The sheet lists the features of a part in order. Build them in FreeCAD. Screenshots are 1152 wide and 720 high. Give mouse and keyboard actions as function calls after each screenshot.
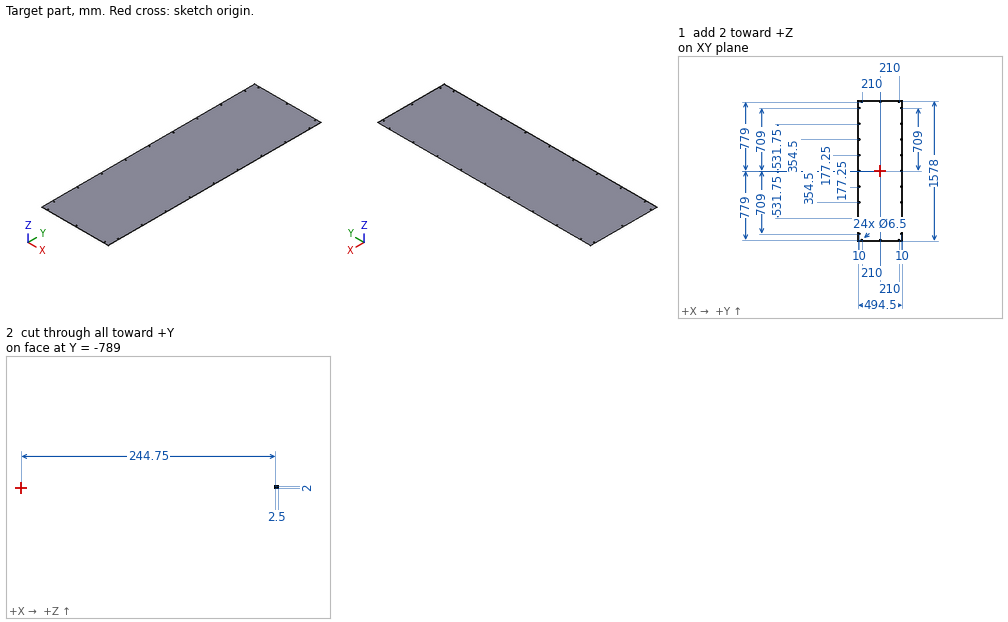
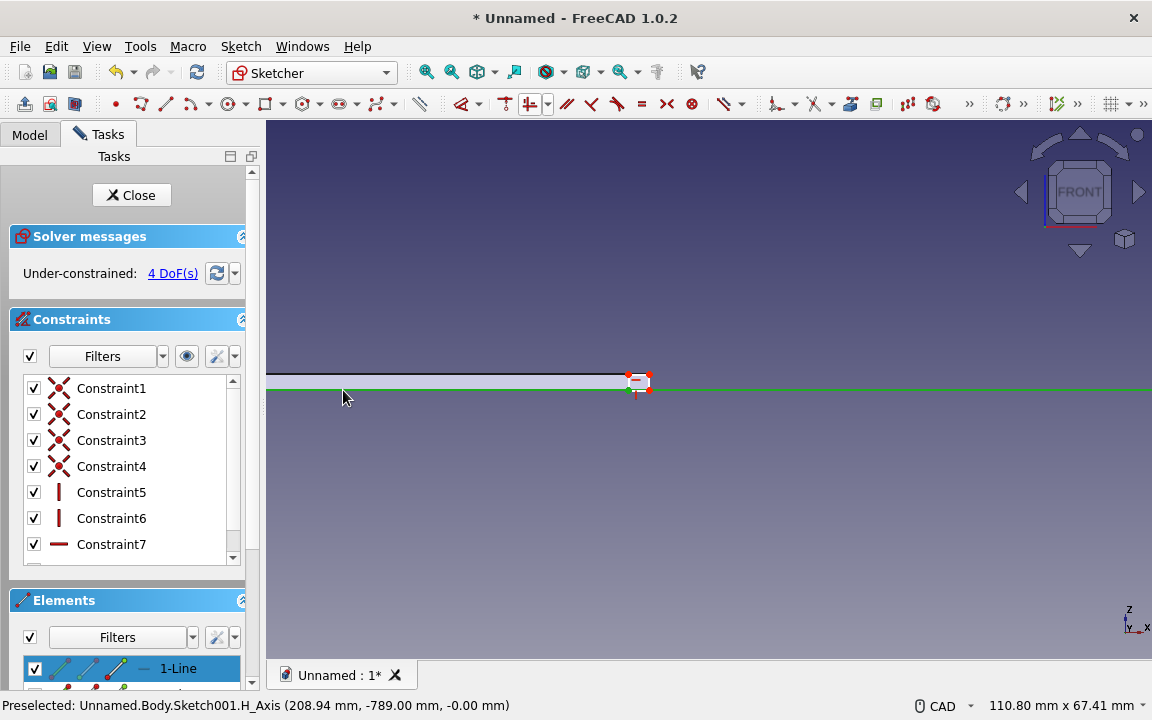
click(505, 104)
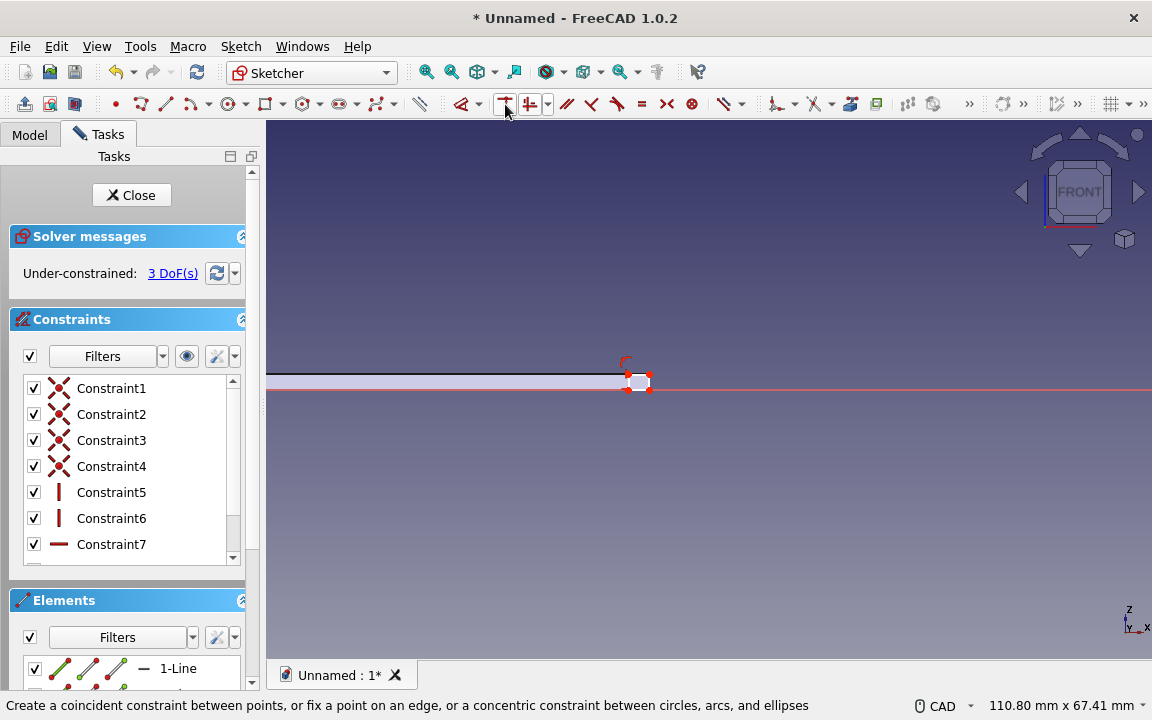
click(460, 104)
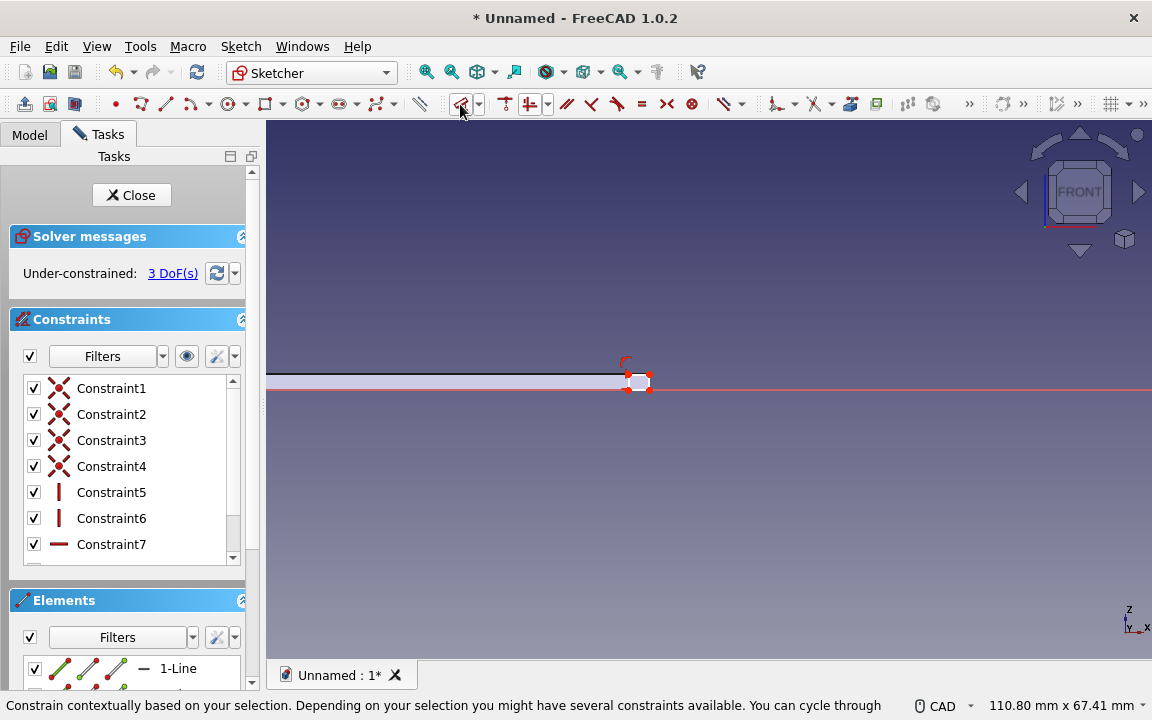
scroll(629, 383, up, 5)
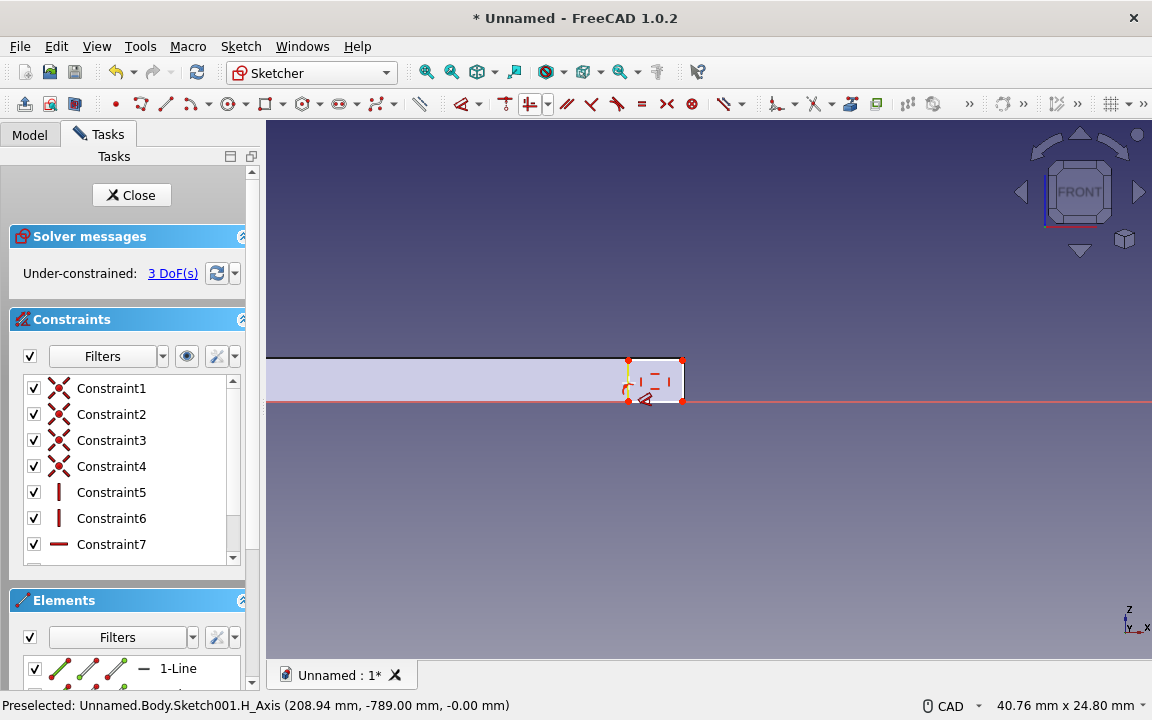
click(628, 381)
click(594, 381)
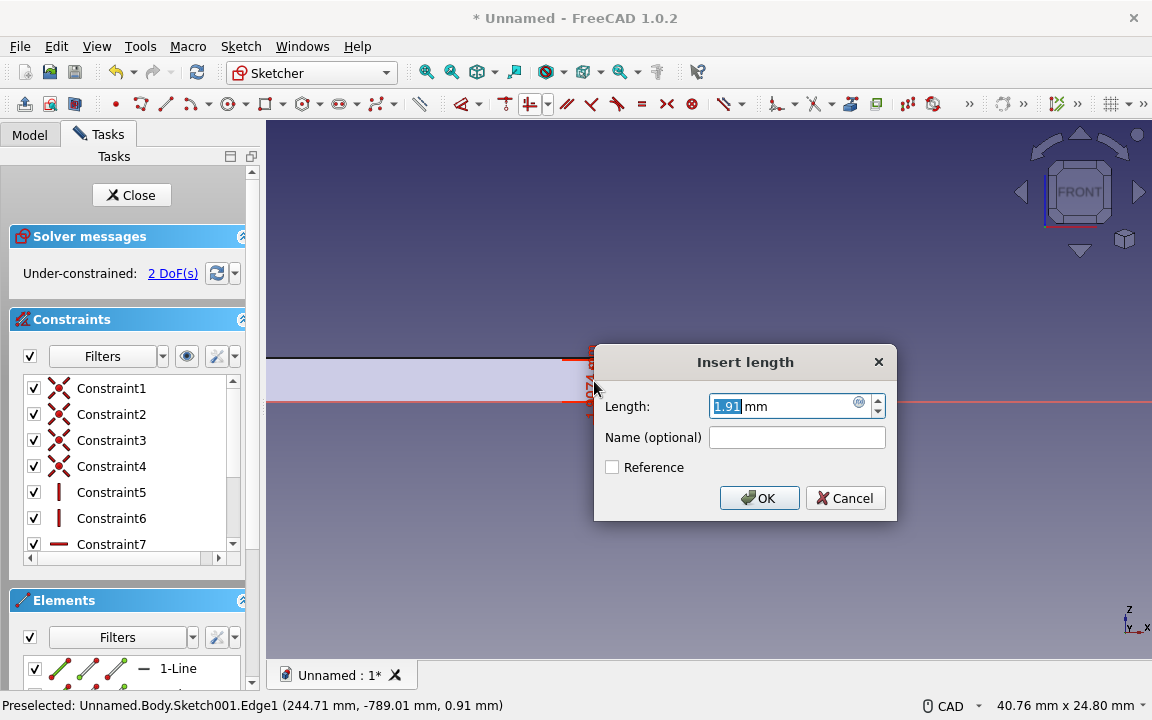
text(2)
key(Return)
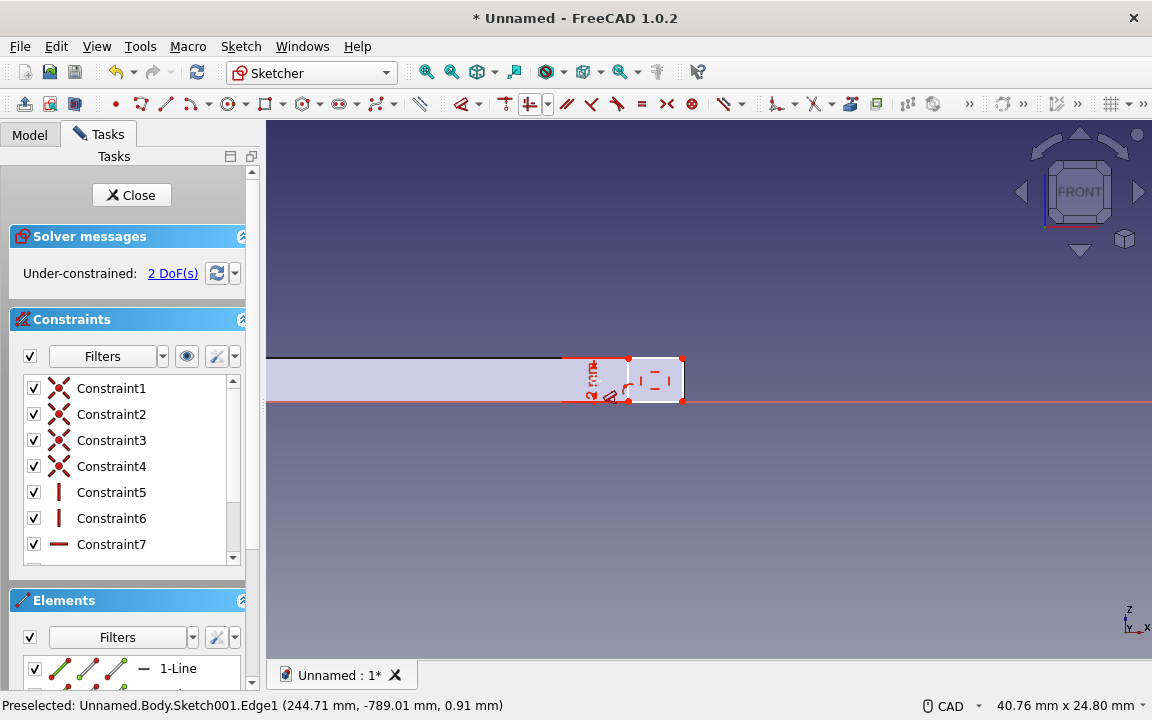
click(645, 402)
click(655, 436)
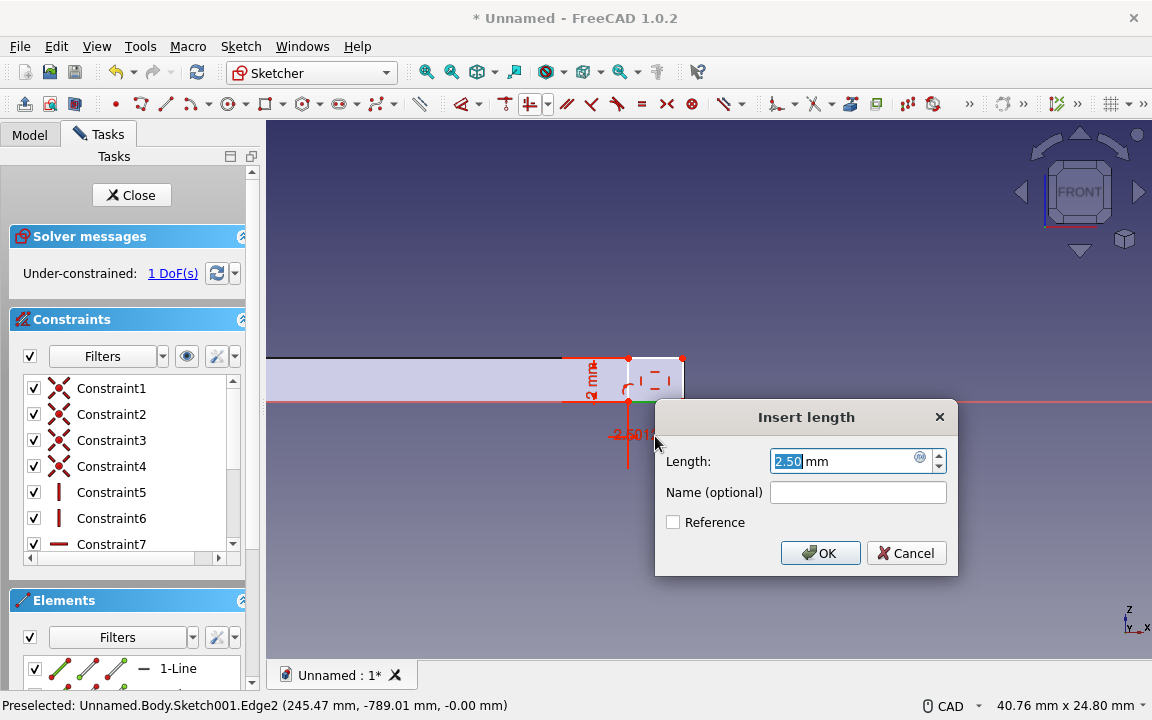
text(2.5)
key(Return)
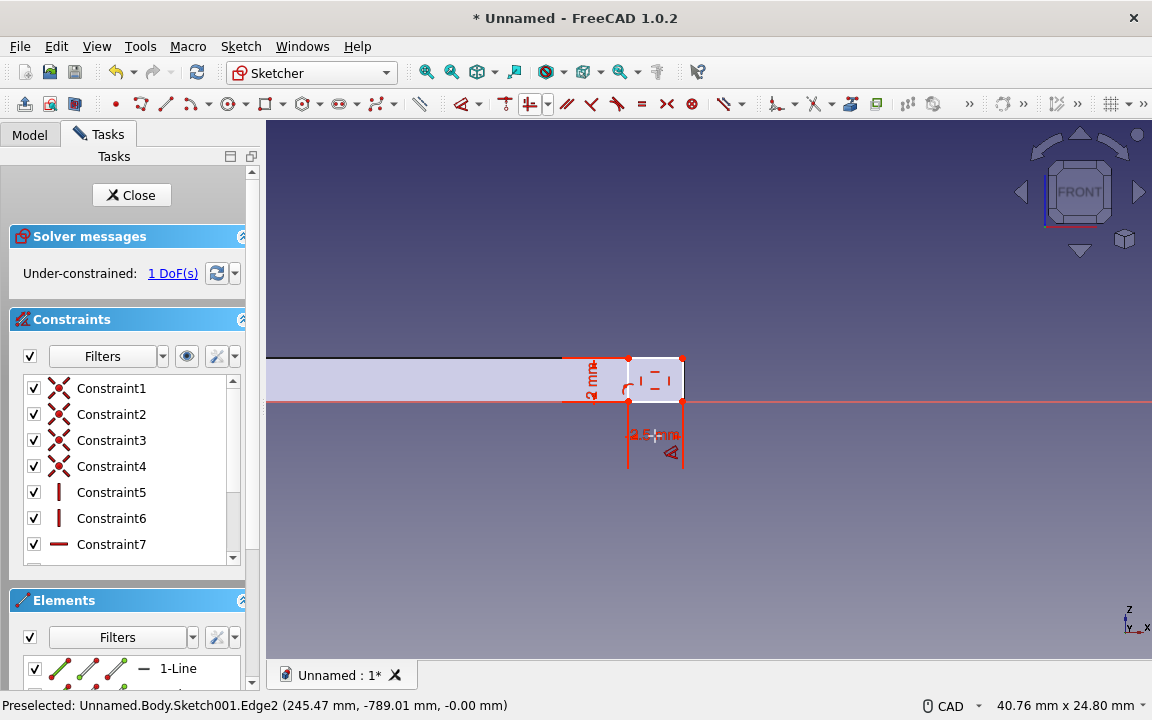
scroll(659, 379, up, 10)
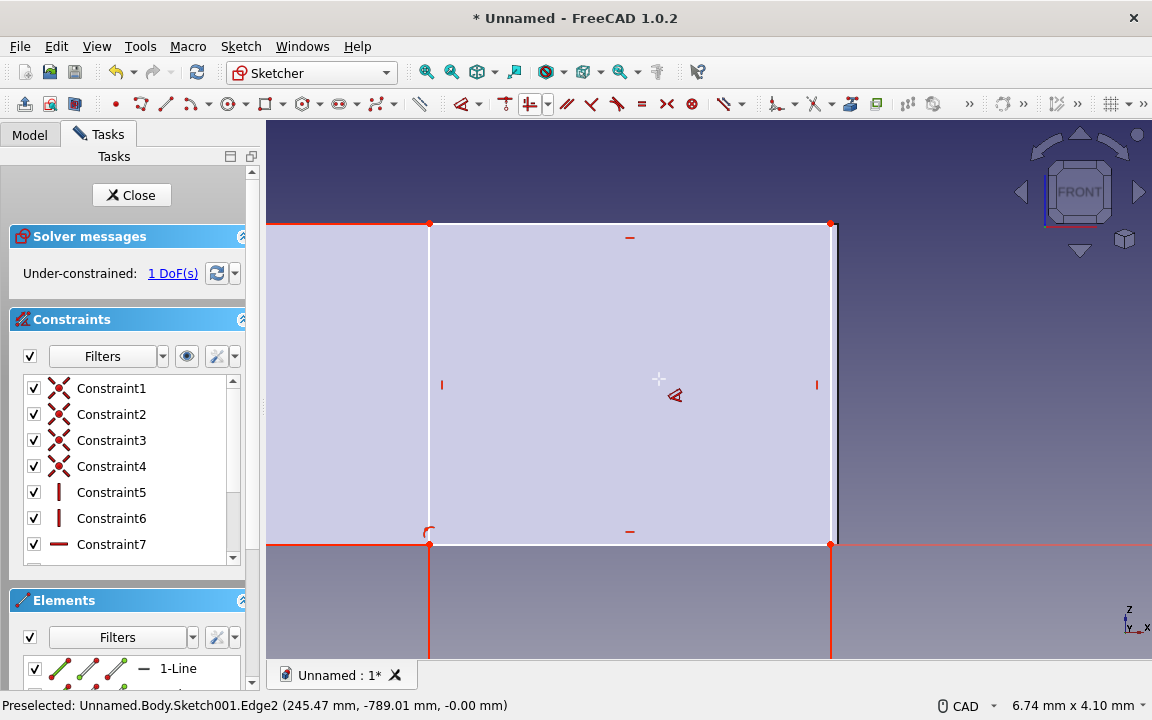
click(429, 224)
click(362, 579)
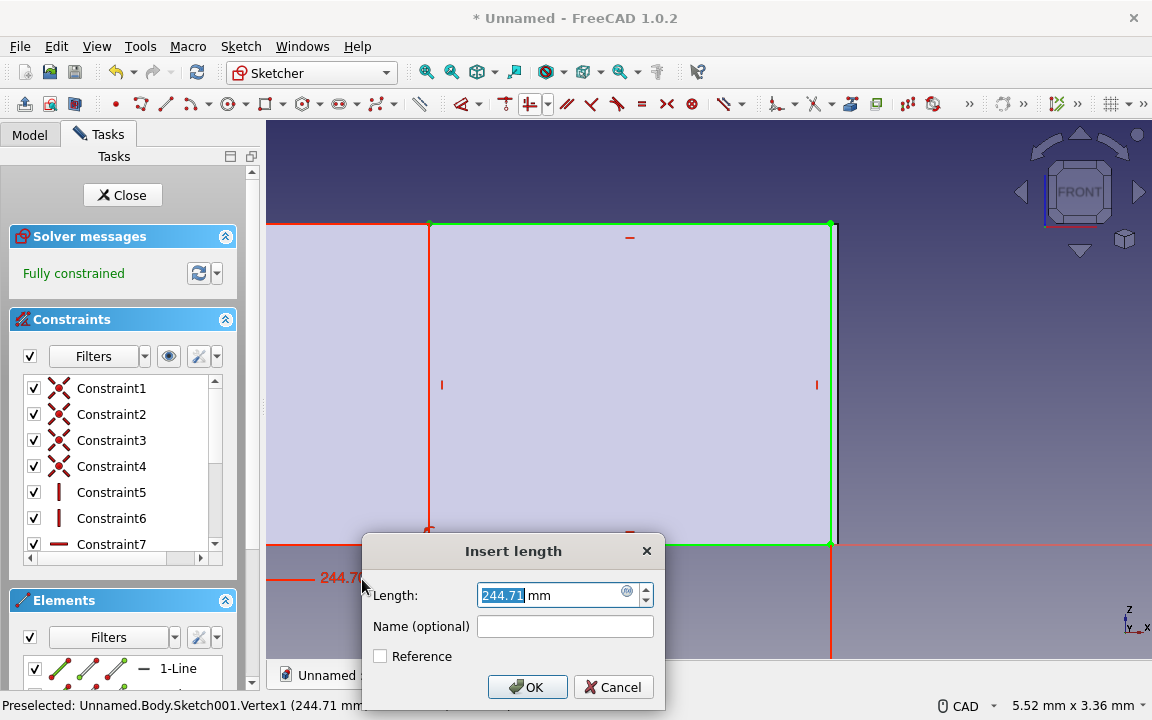
text(244.75)
key(Return)
key(Escape)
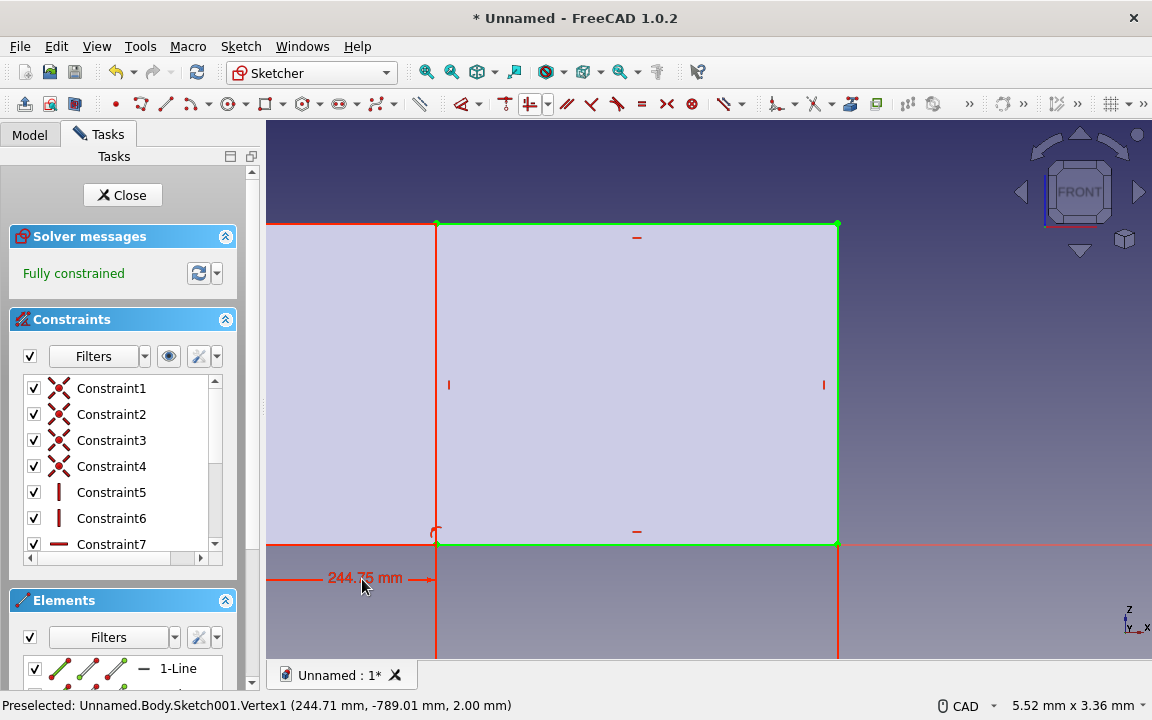
click(123, 195)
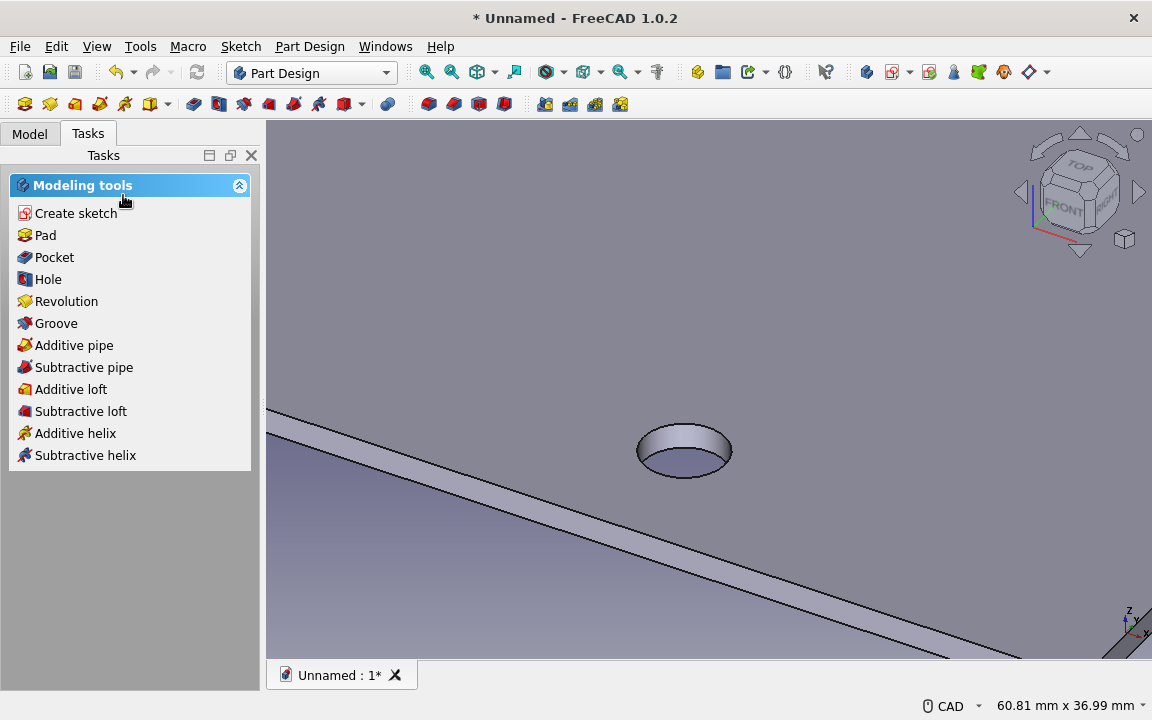
click(194, 104)